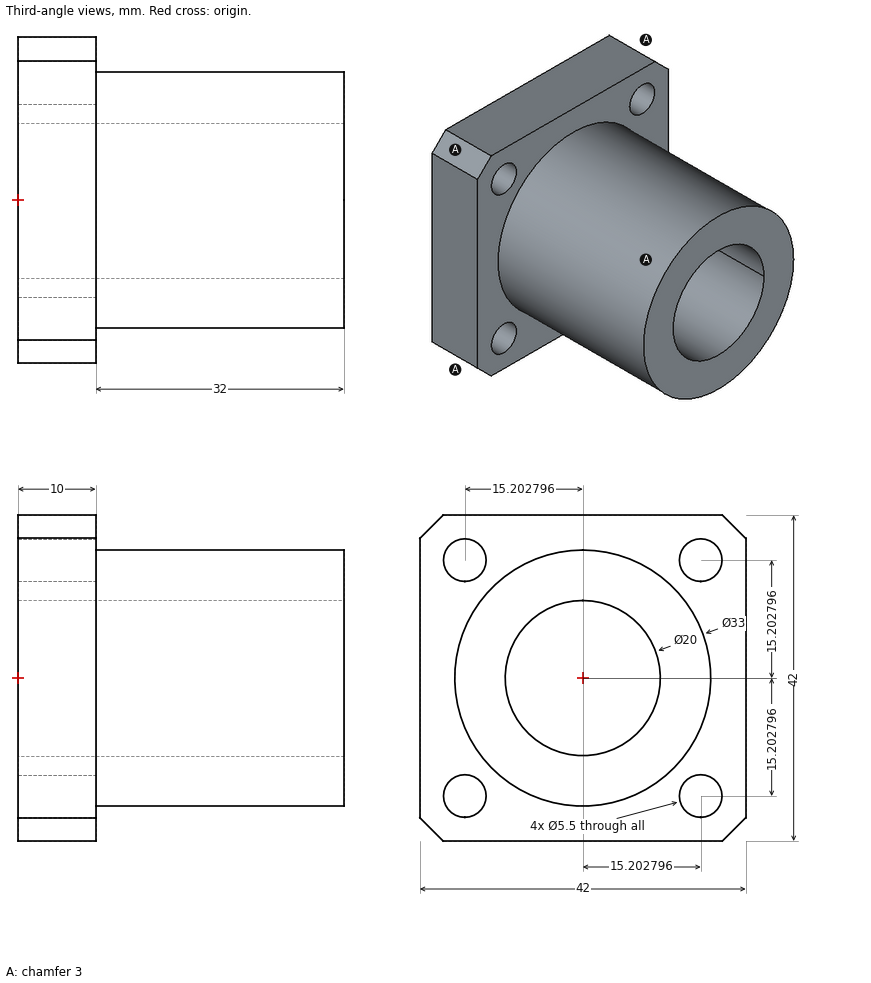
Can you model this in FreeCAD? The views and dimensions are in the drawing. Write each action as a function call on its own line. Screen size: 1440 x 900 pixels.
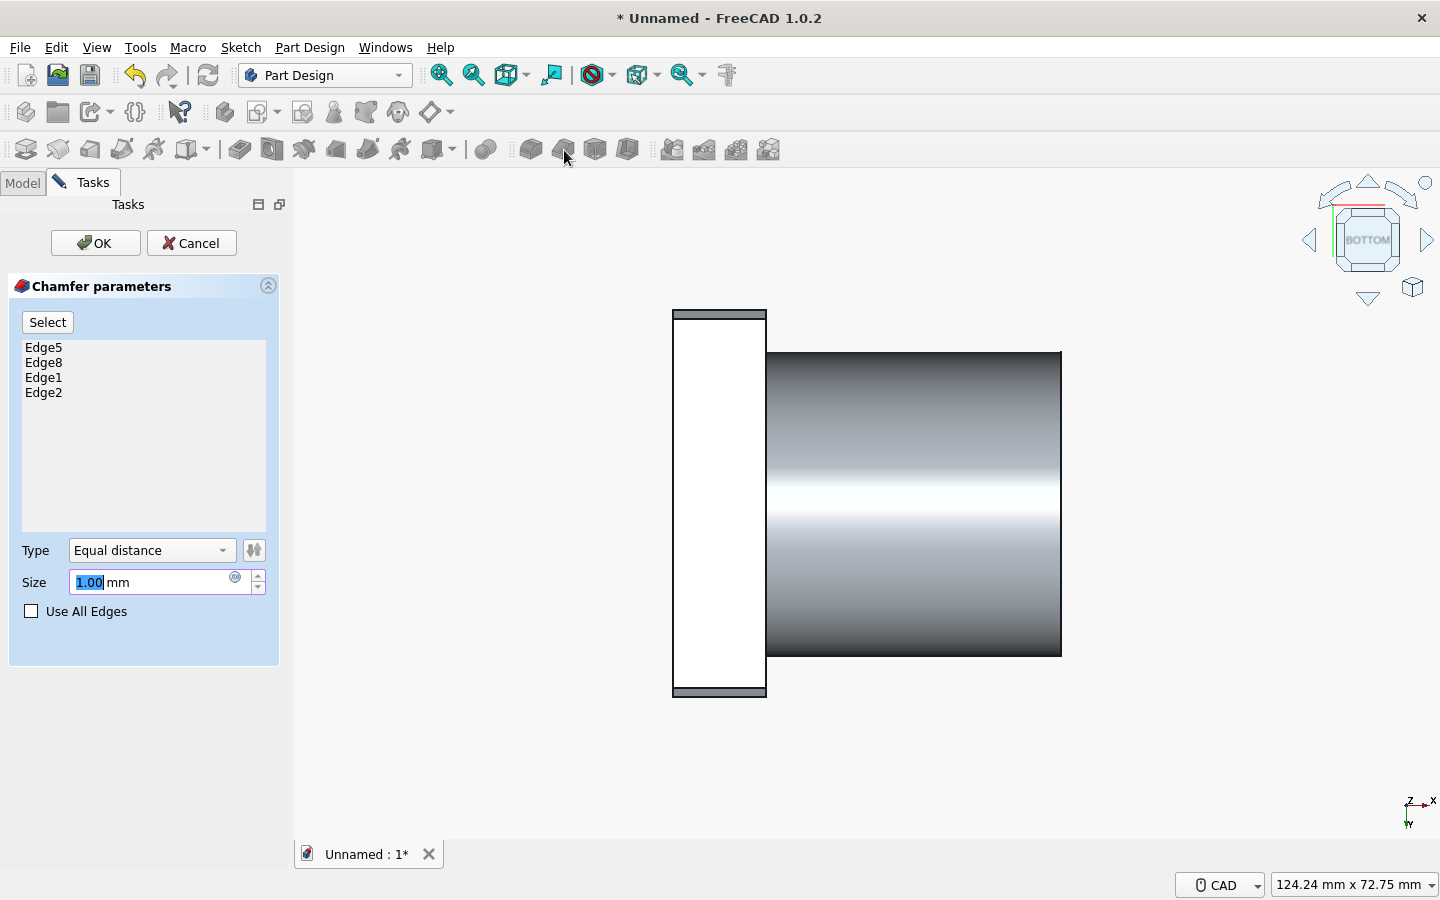
text(3)
key(Tab)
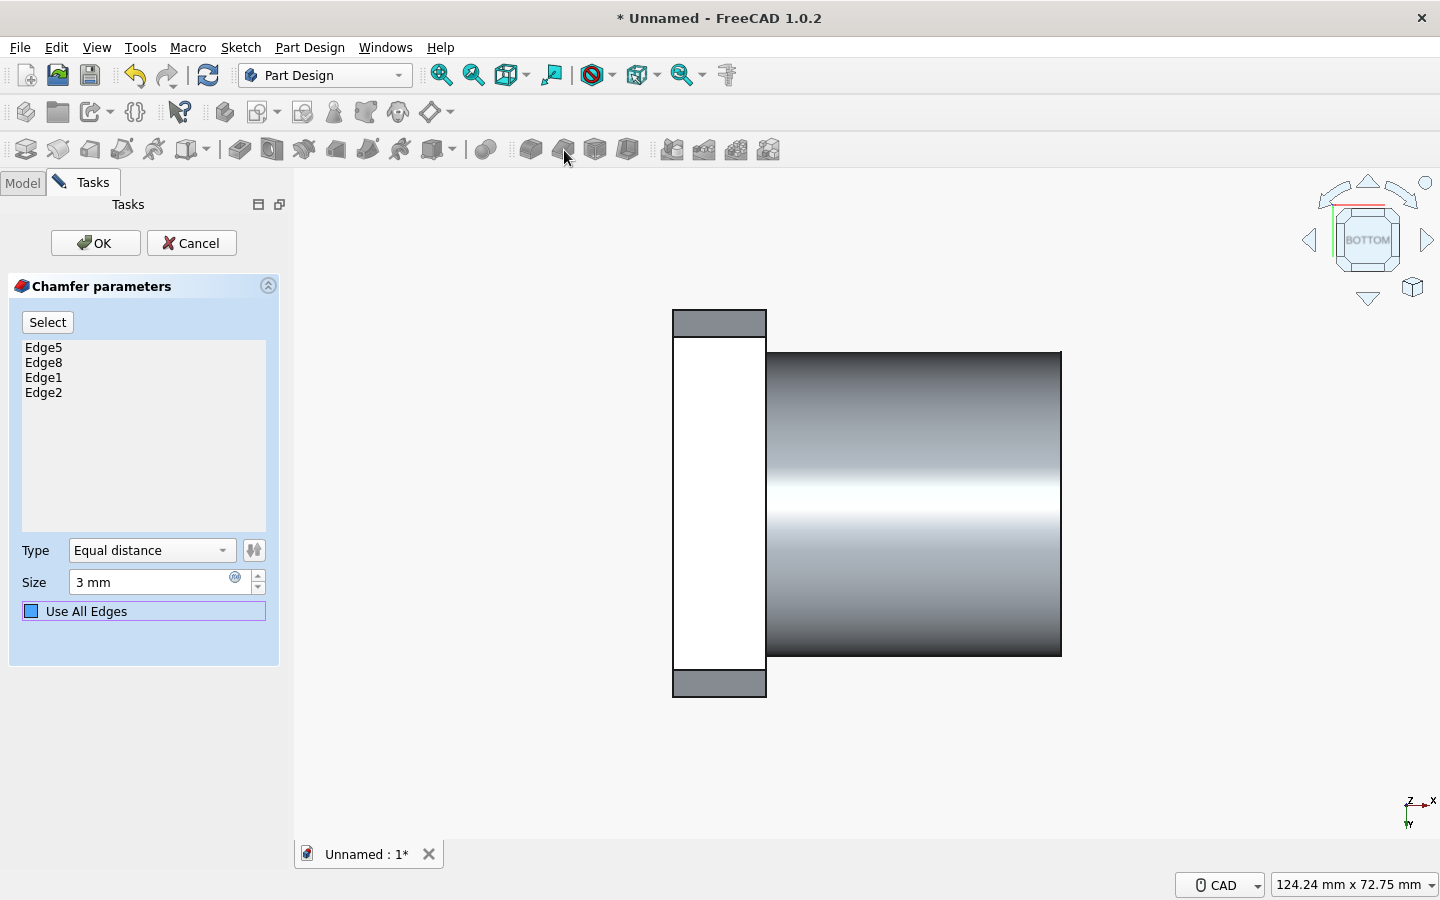
click(96, 243)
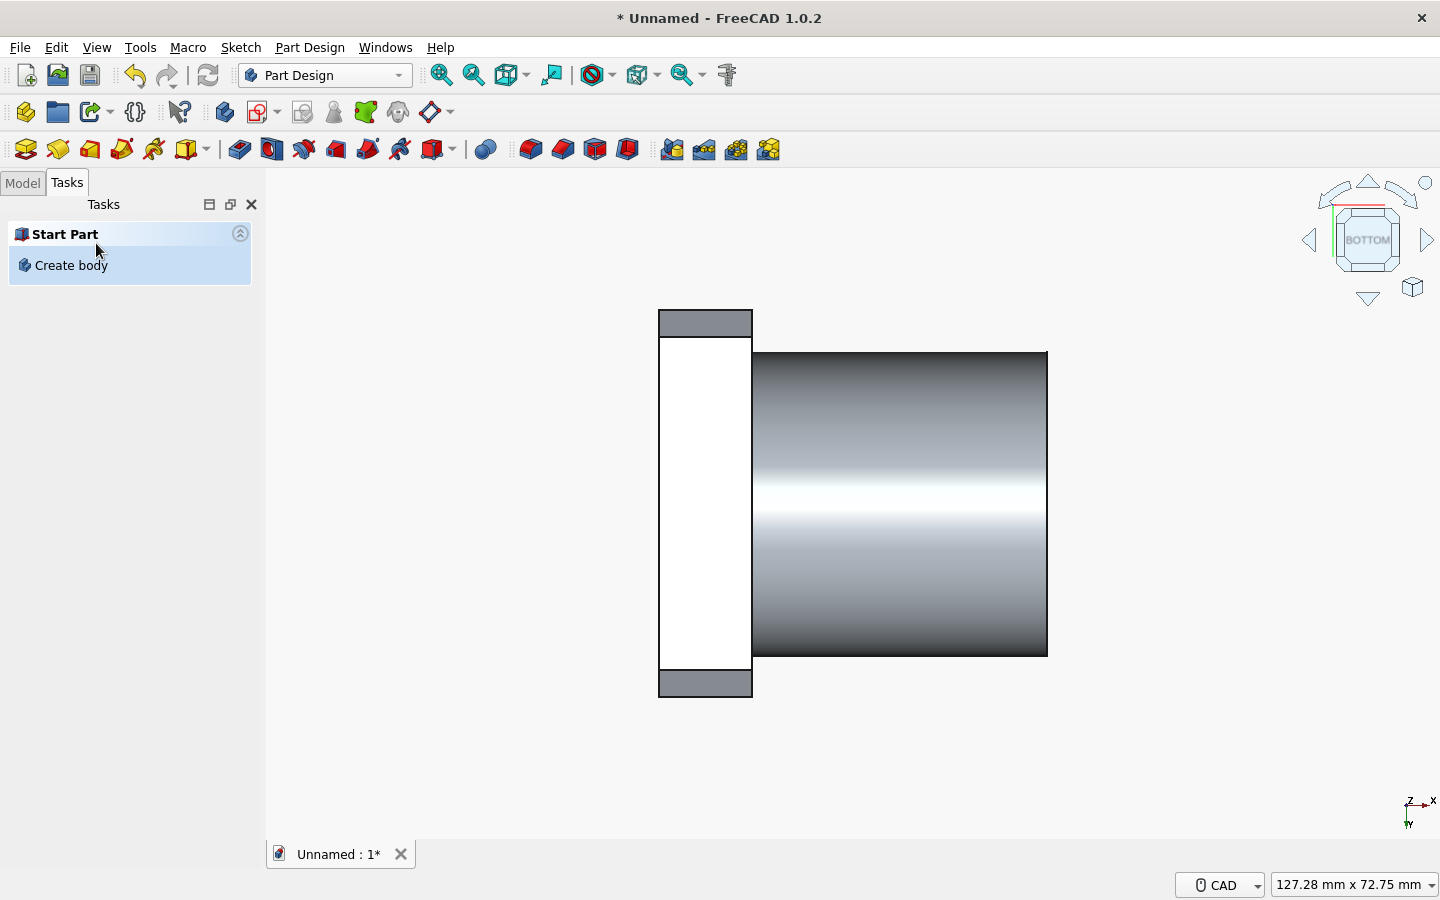
key(0)